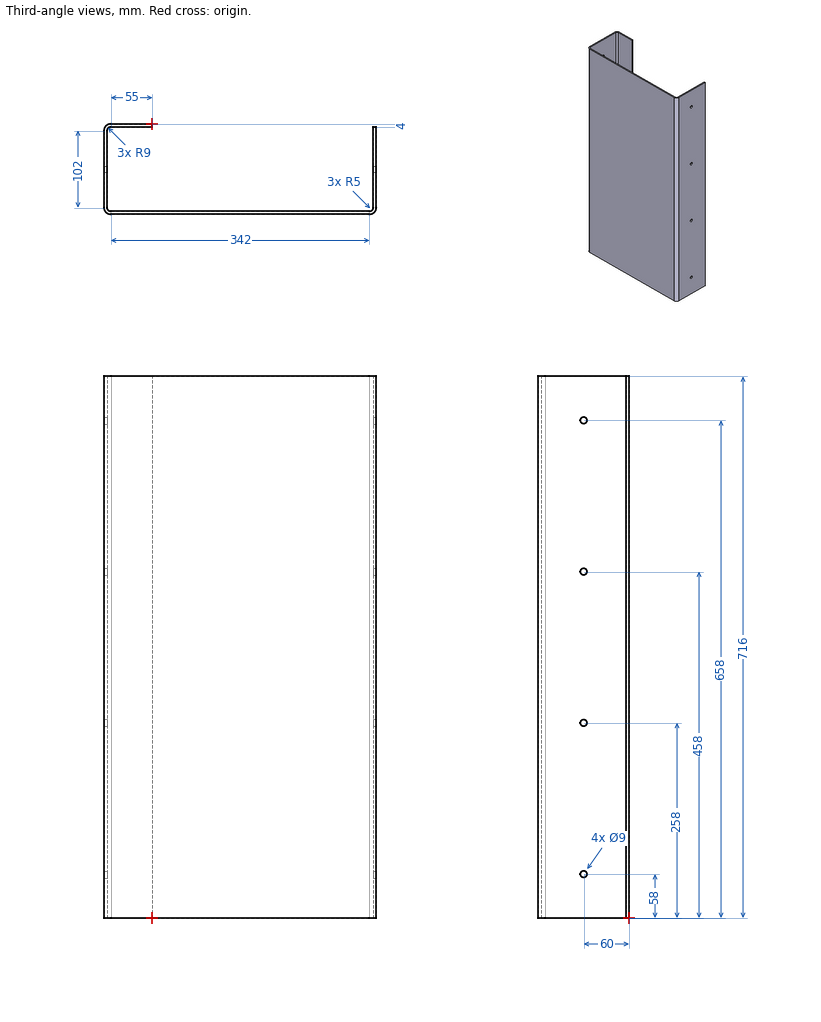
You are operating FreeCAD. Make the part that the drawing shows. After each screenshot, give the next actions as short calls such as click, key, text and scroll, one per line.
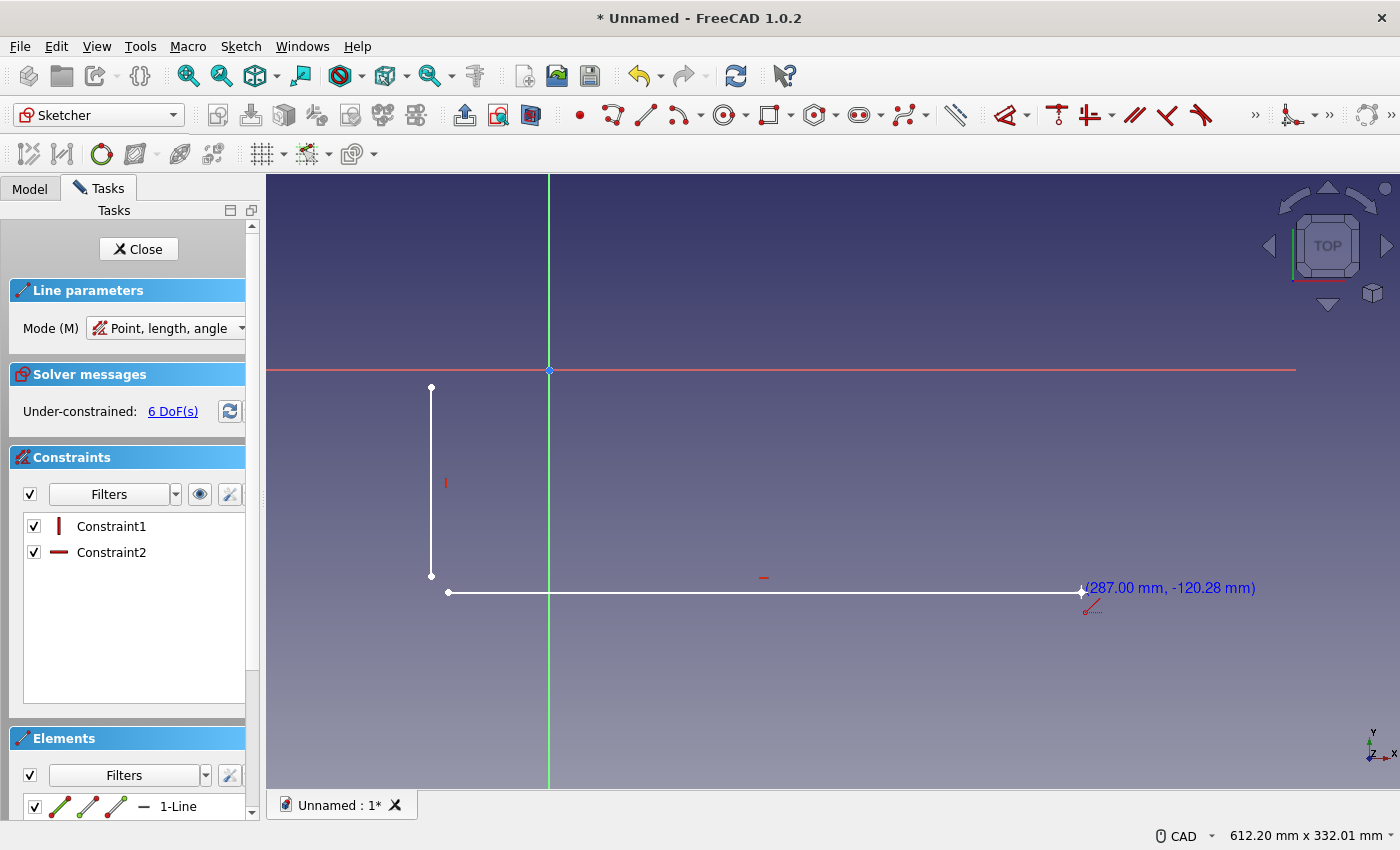
click(613, 116)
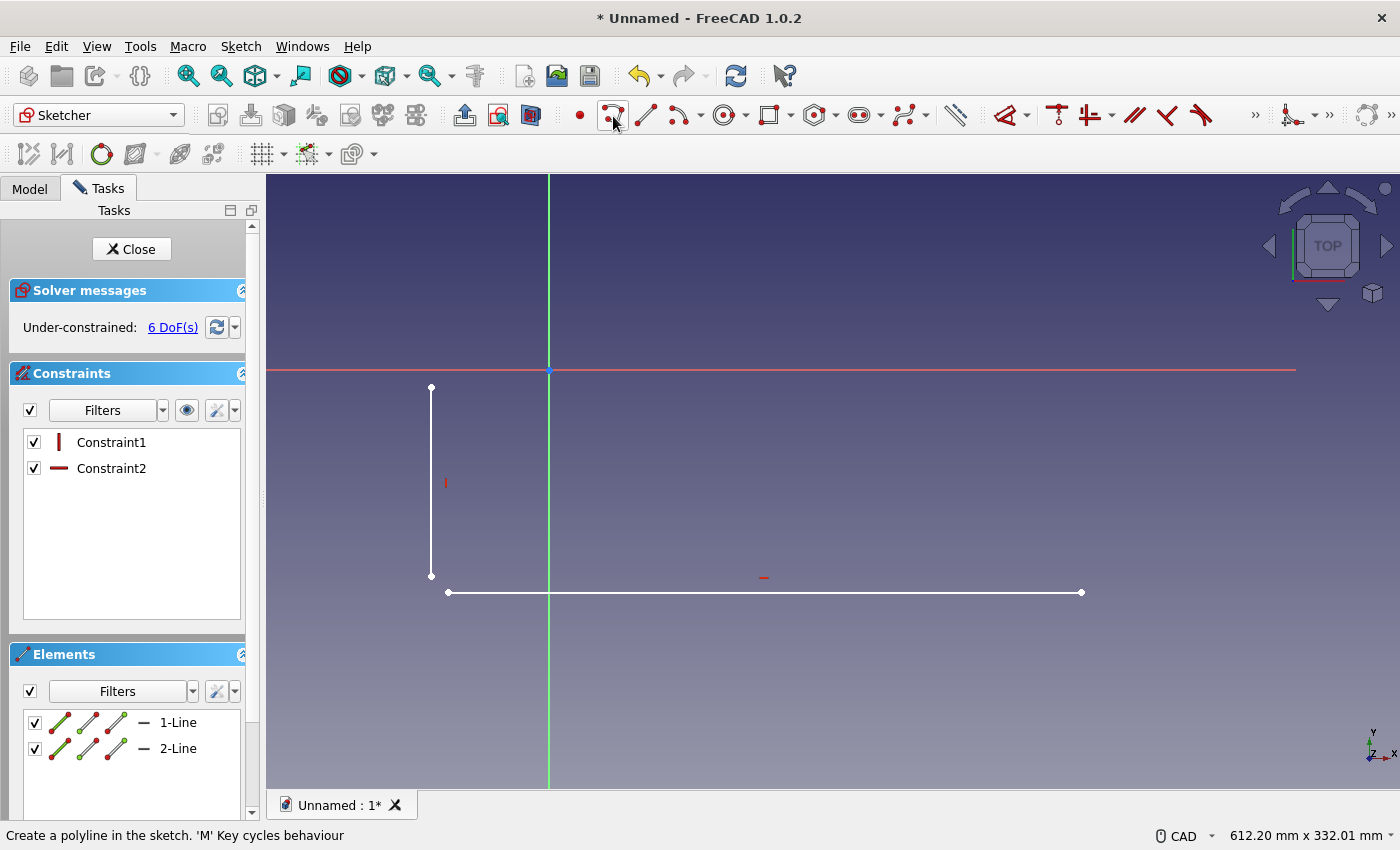
click(1098, 576)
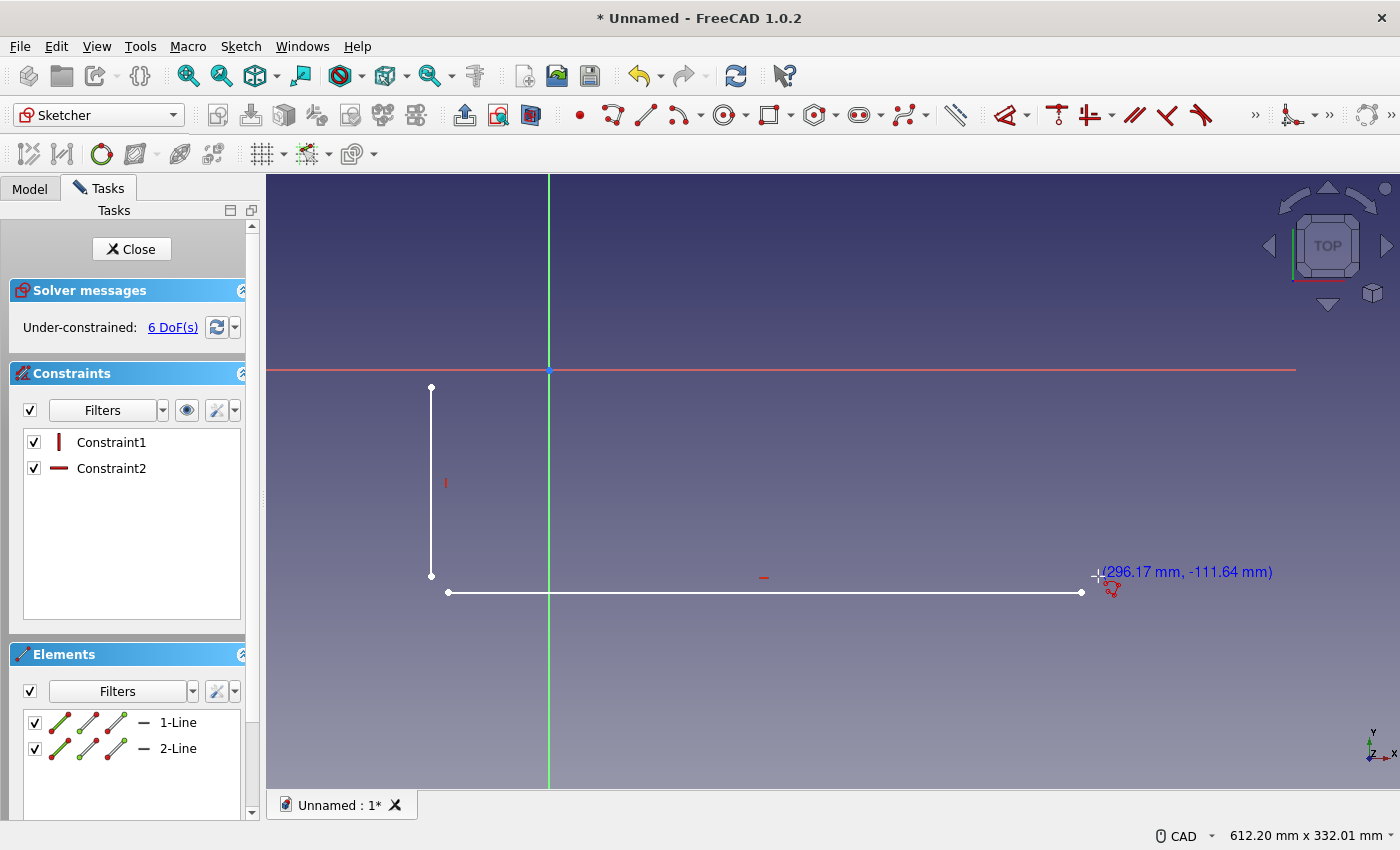
scroll(1098, 378, up, 4)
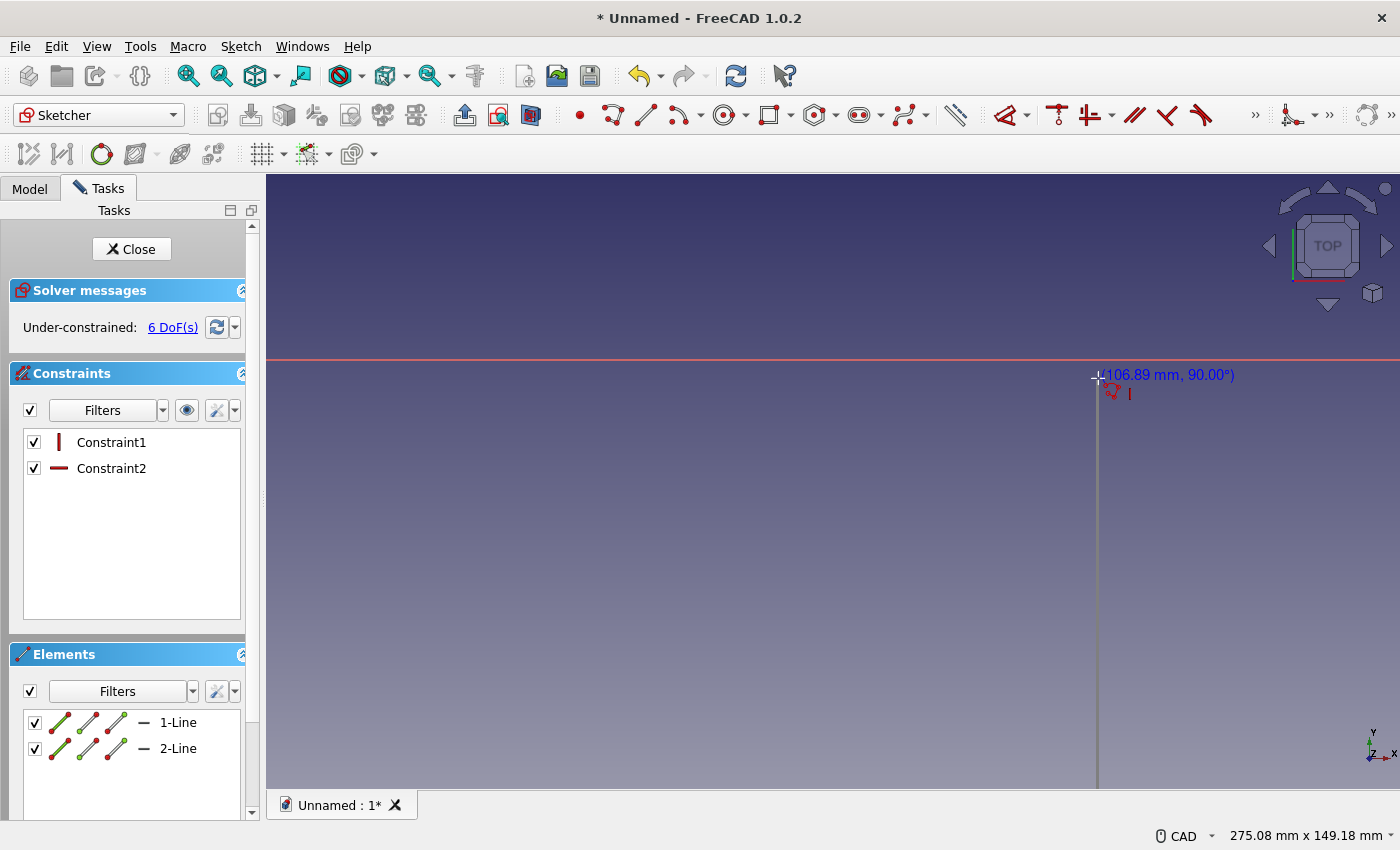
click(1097, 377)
click(1080, 377)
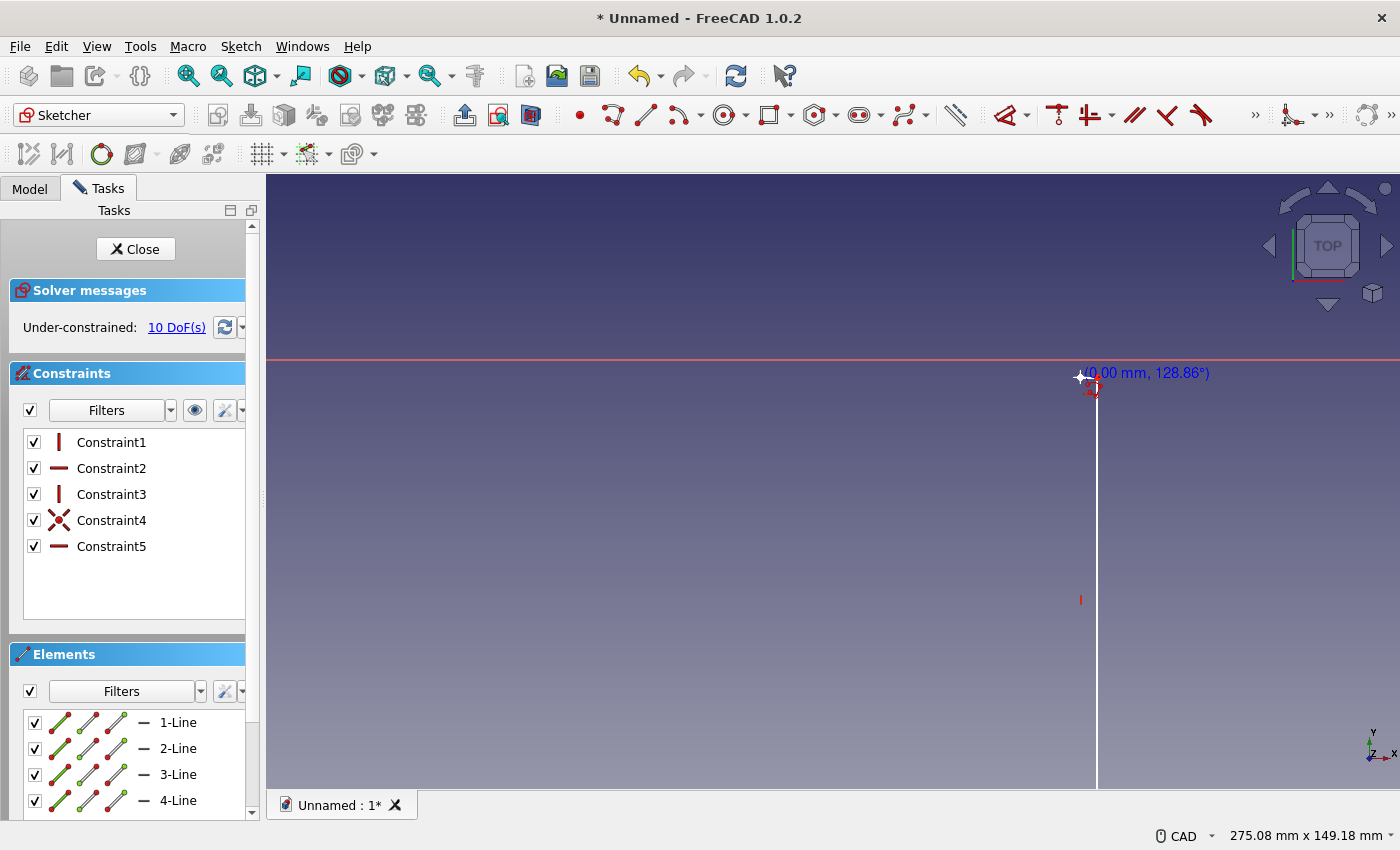
scroll(1099, 379, down, 4)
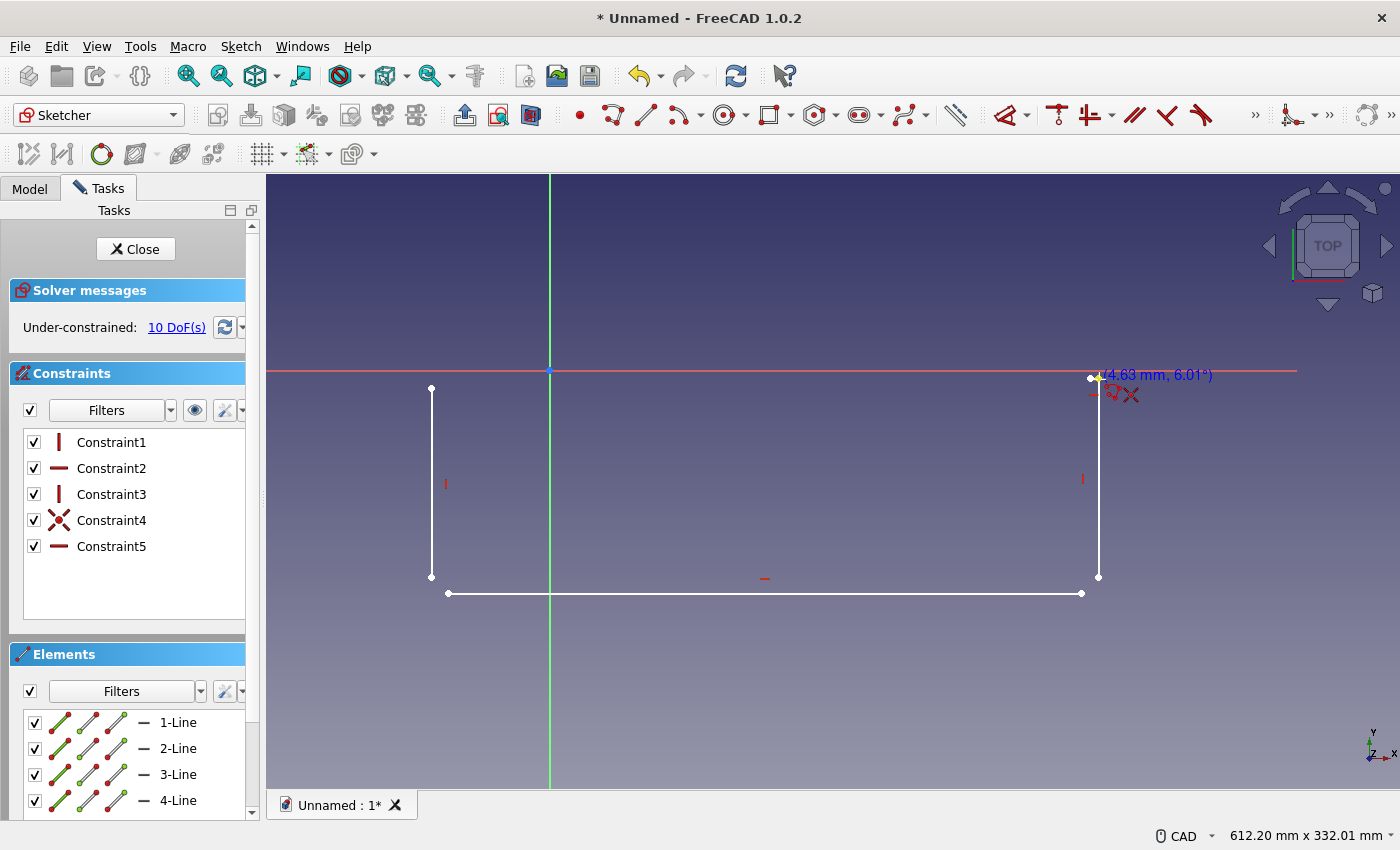
scroll(1091, 576, up, 4)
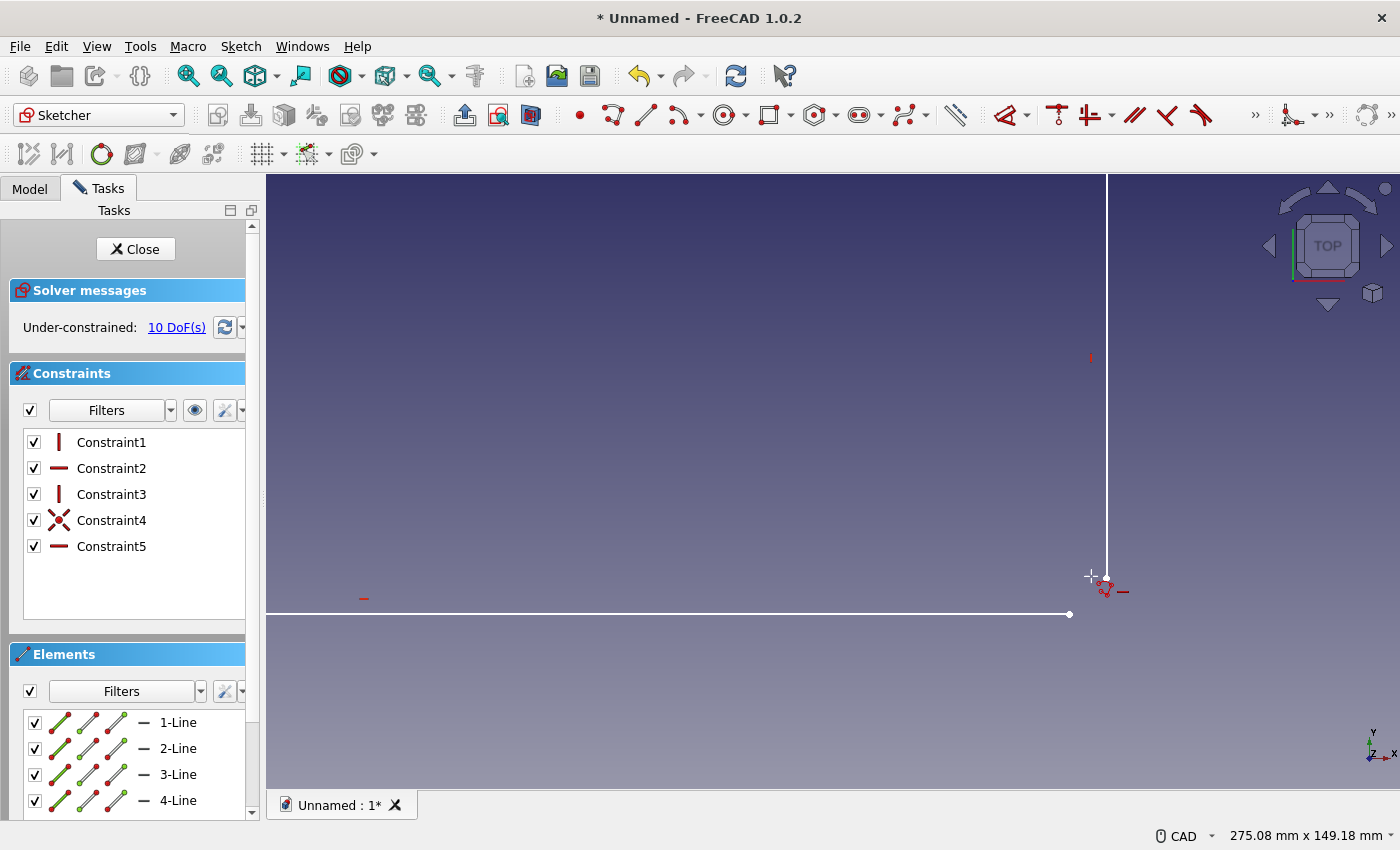
click(1090, 576)
right_click(1090, 576)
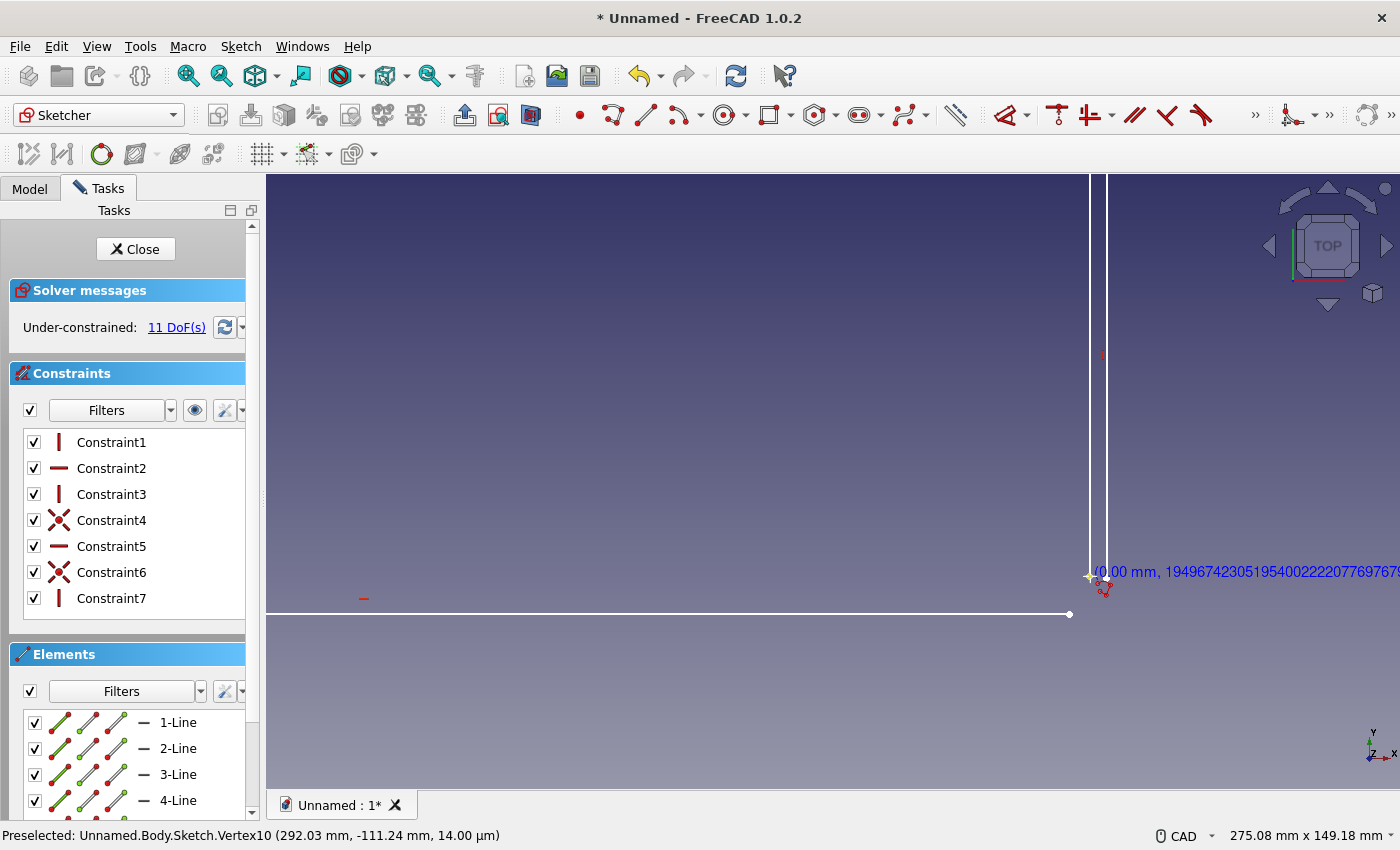
click(646, 116)